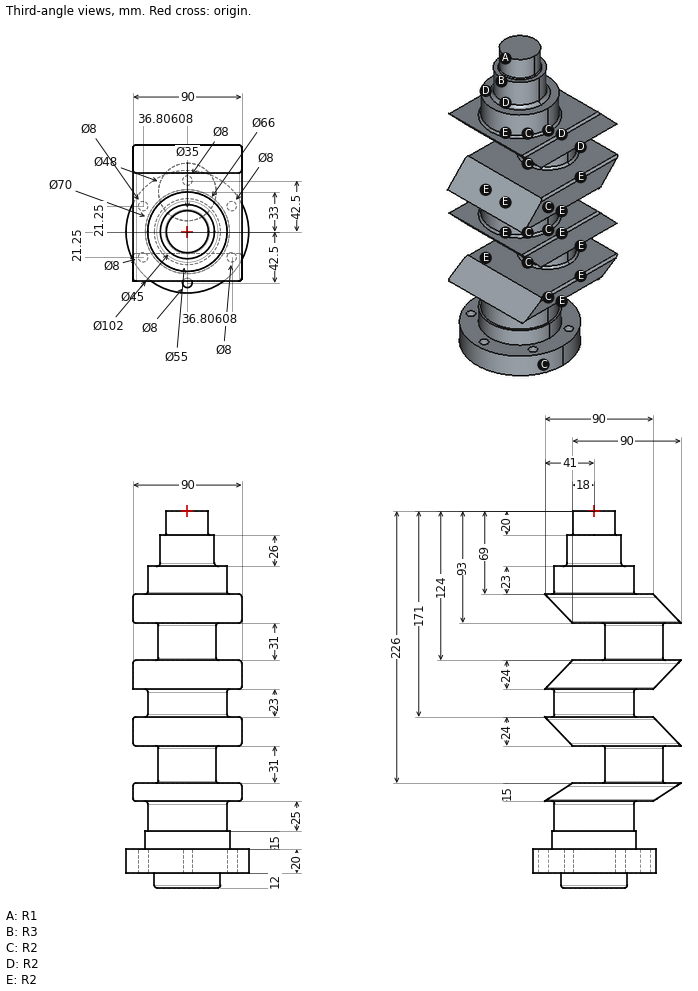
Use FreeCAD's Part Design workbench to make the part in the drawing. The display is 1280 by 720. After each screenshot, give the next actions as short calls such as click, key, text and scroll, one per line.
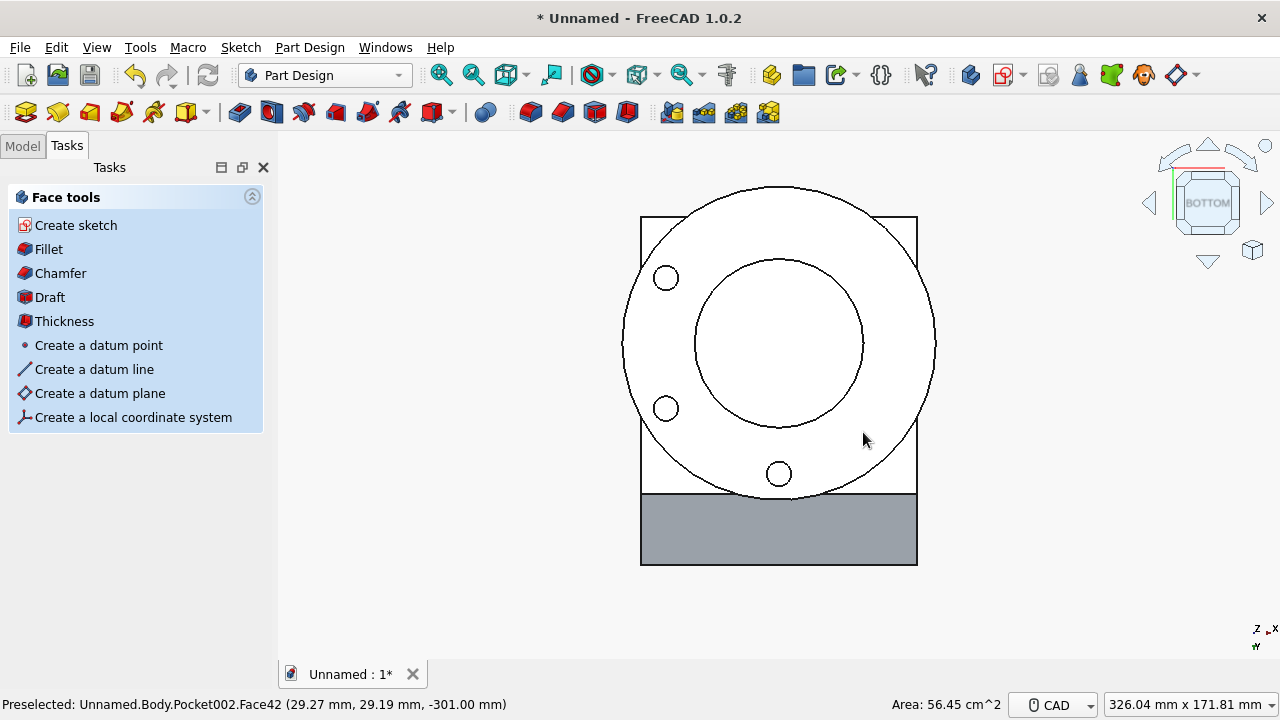
click(1004, 76)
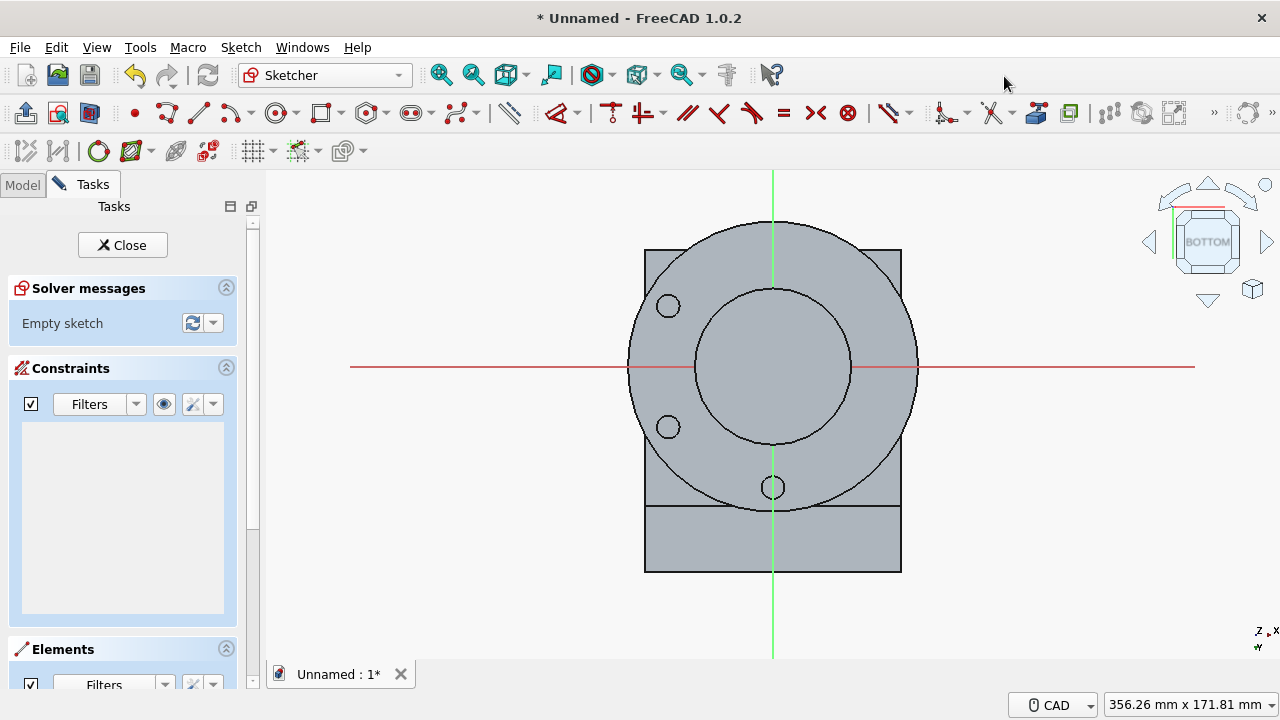
click(90, 114)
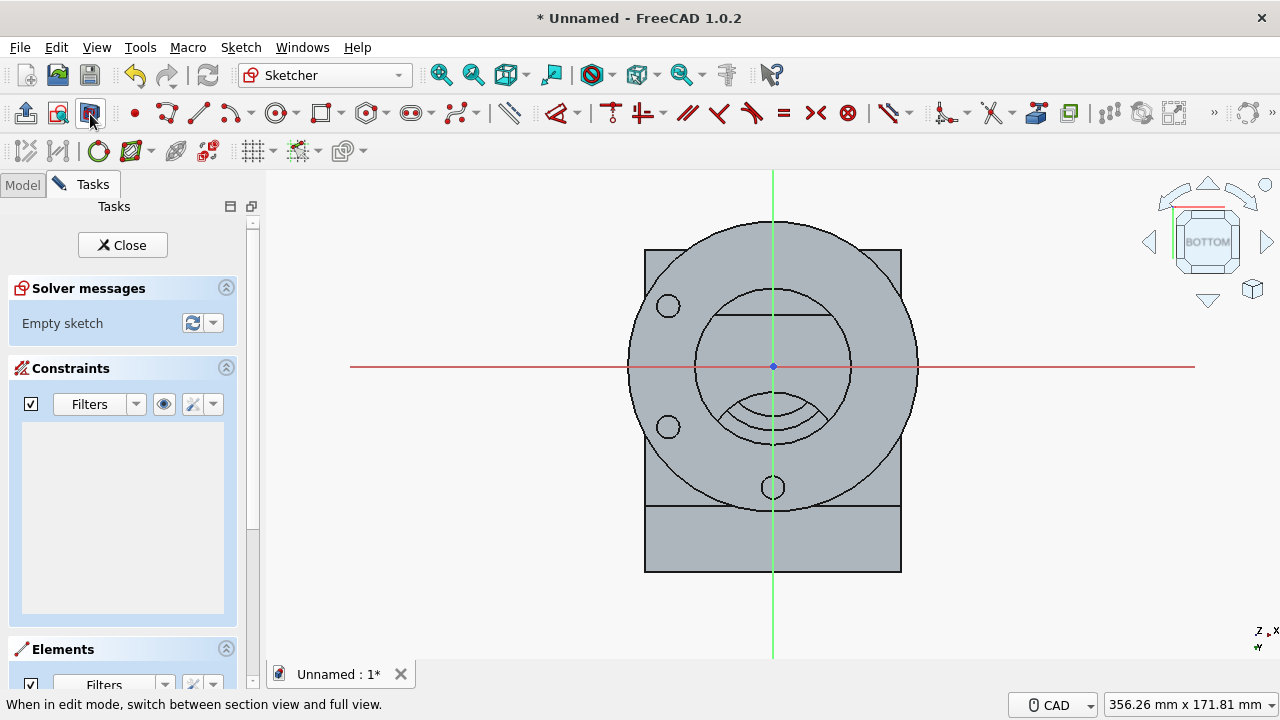
scroll(779, 232, up, 13)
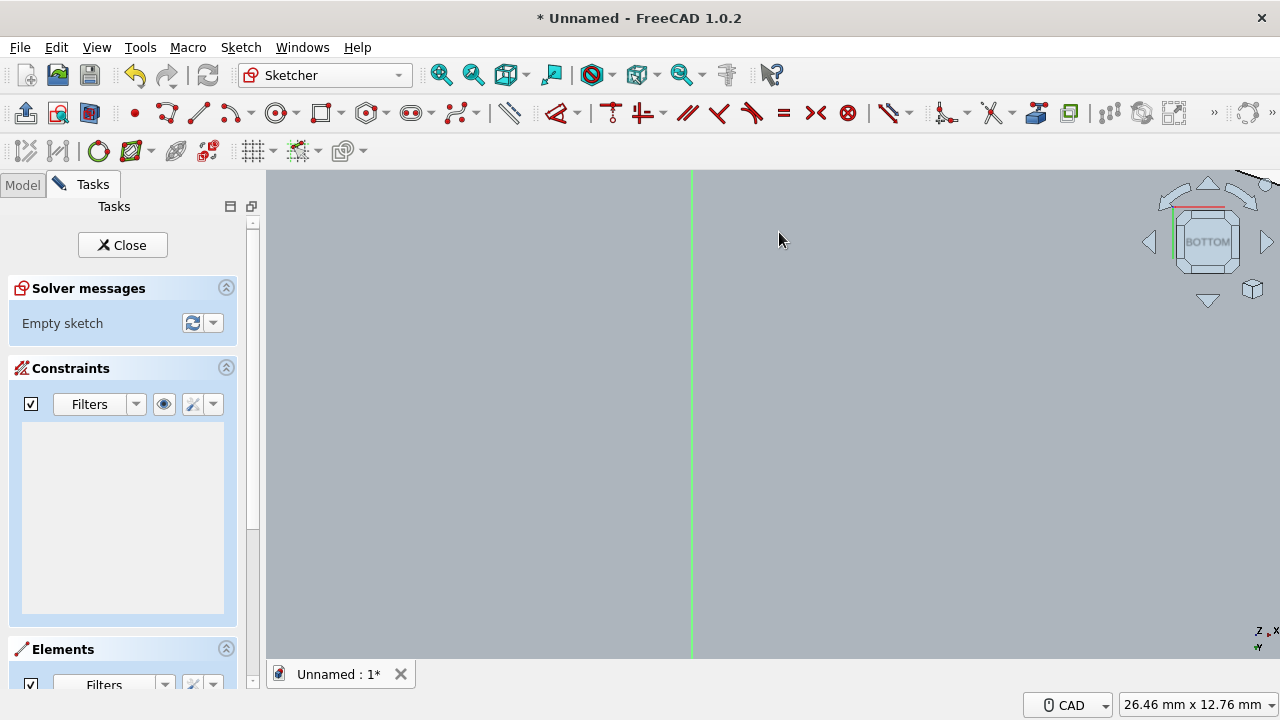
click(276, 114)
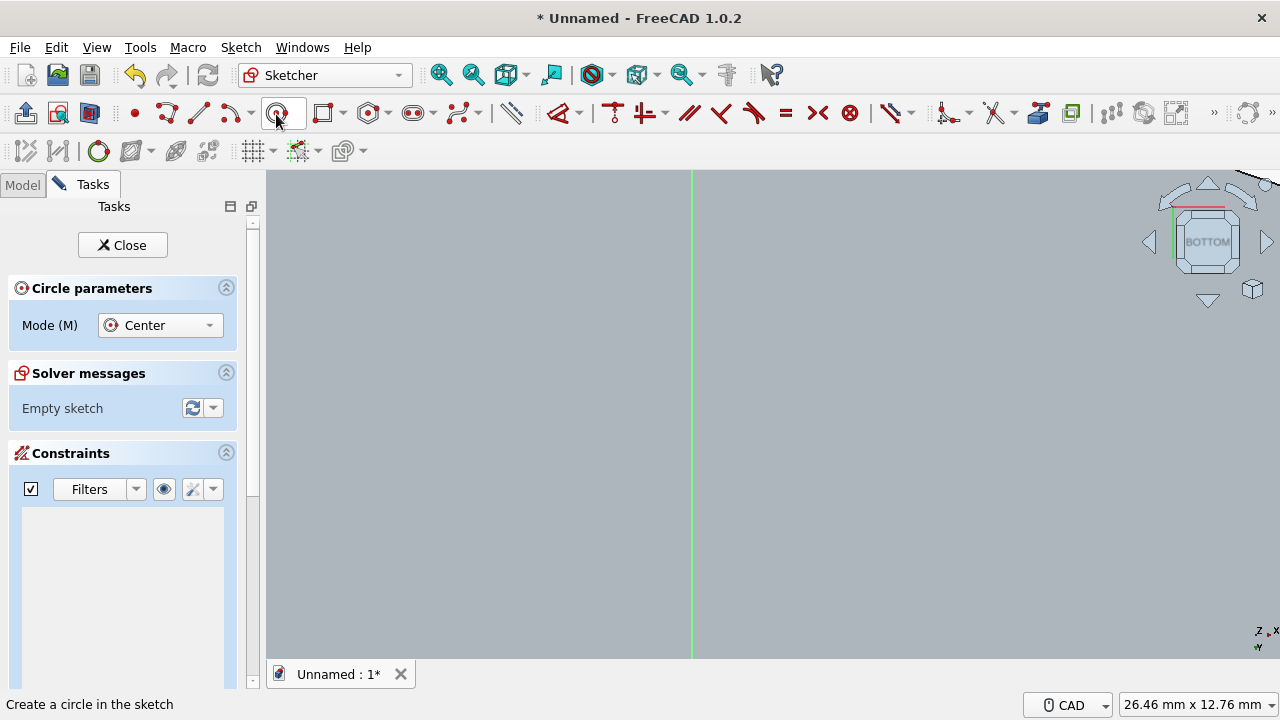
click(692, 414)
move(801, 306)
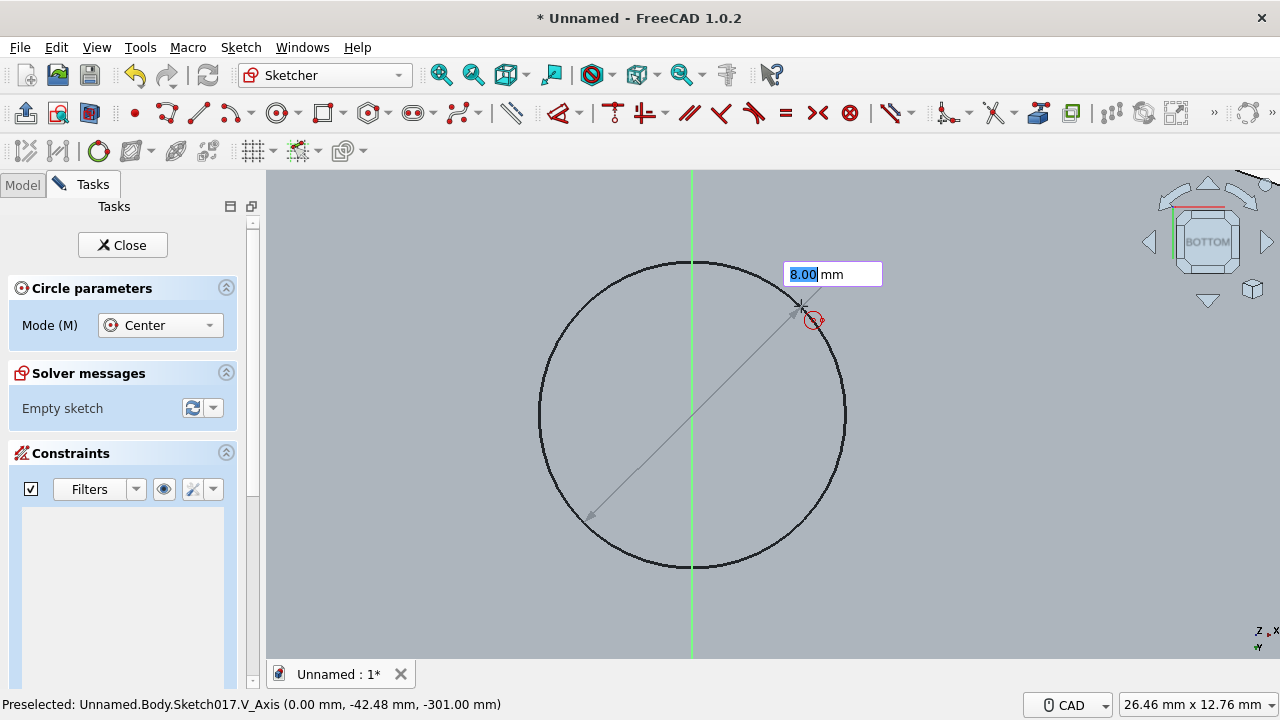
text(8)
key(Return)
key(Escape)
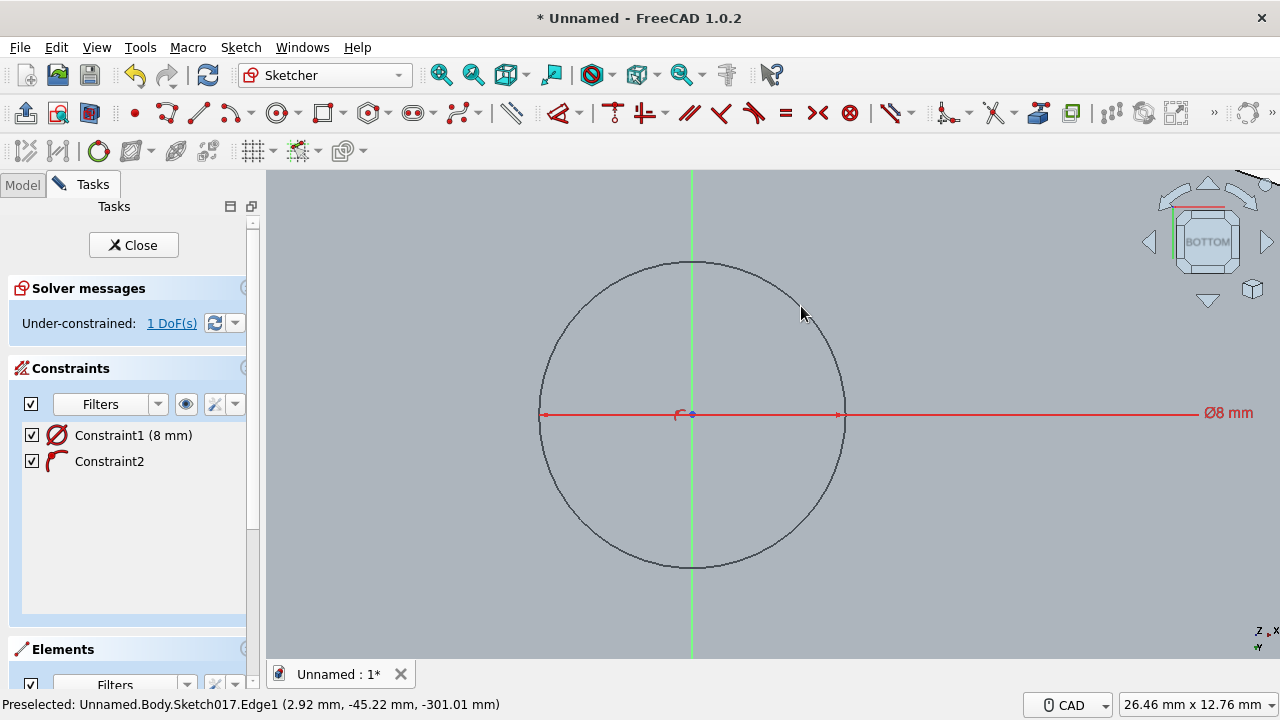
click(558, 114)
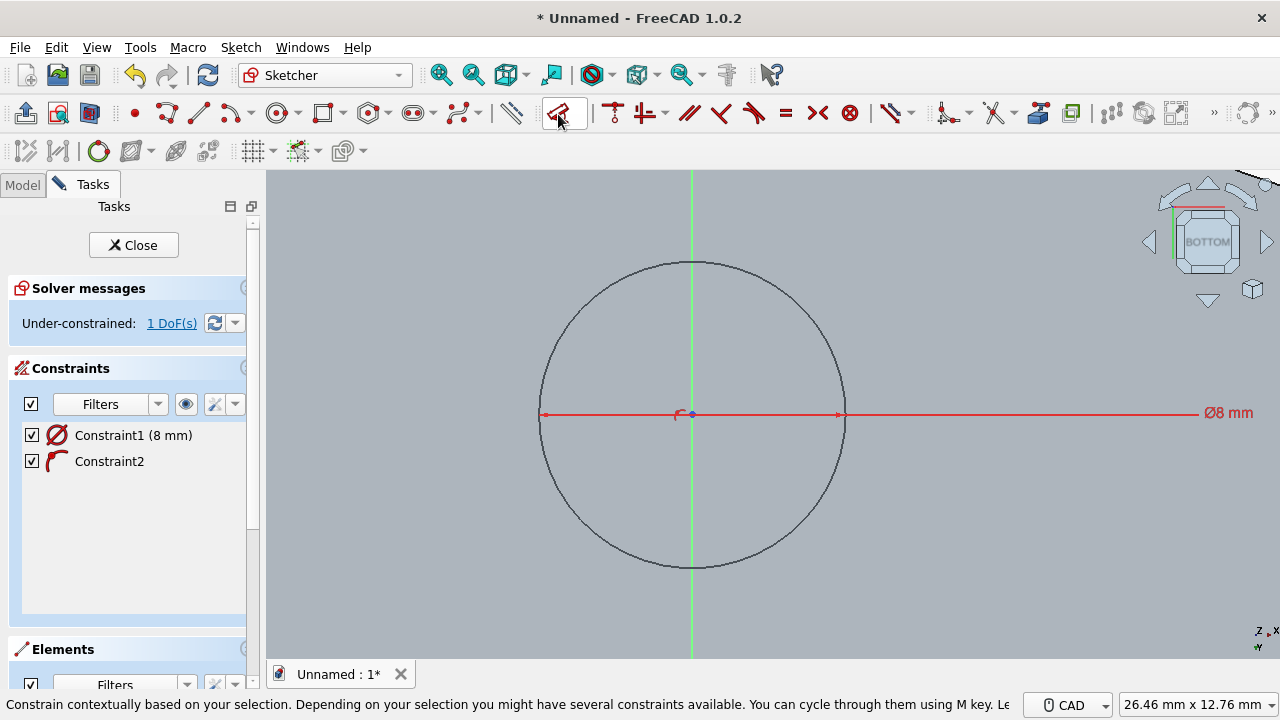
click(692, 415)
click(726, 523)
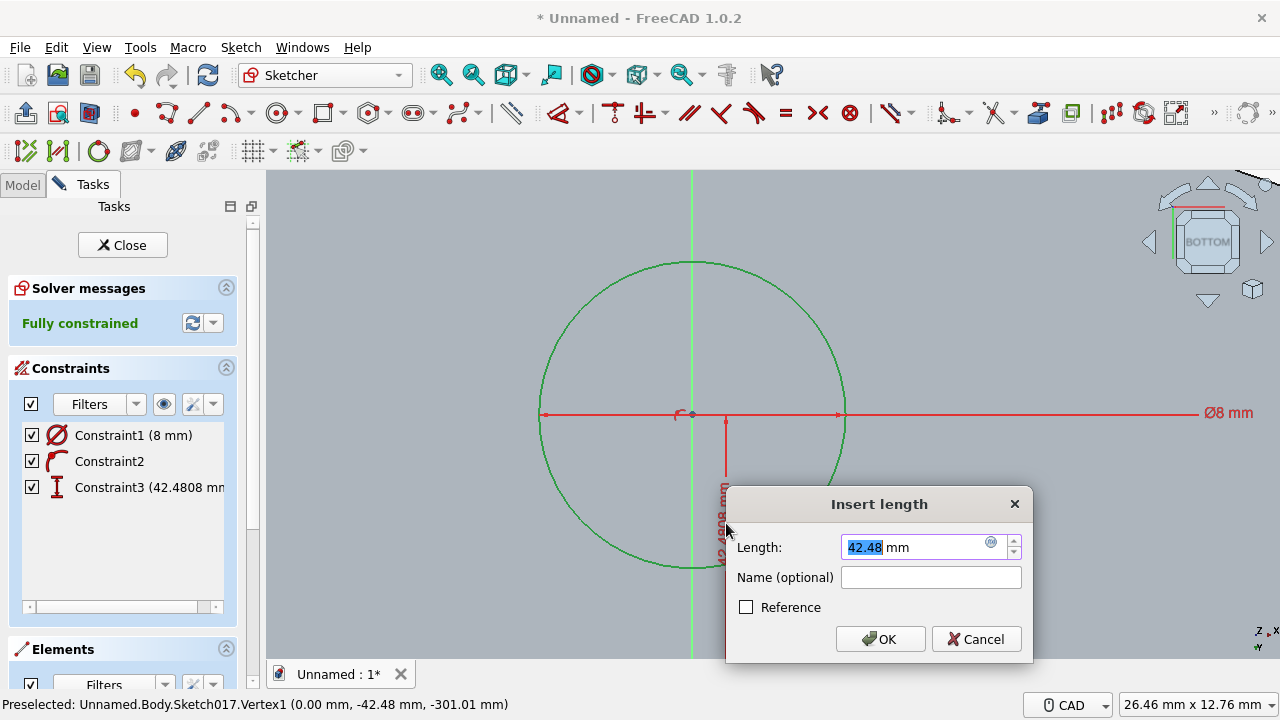
text(42.5)
key(Return)
key(Escape)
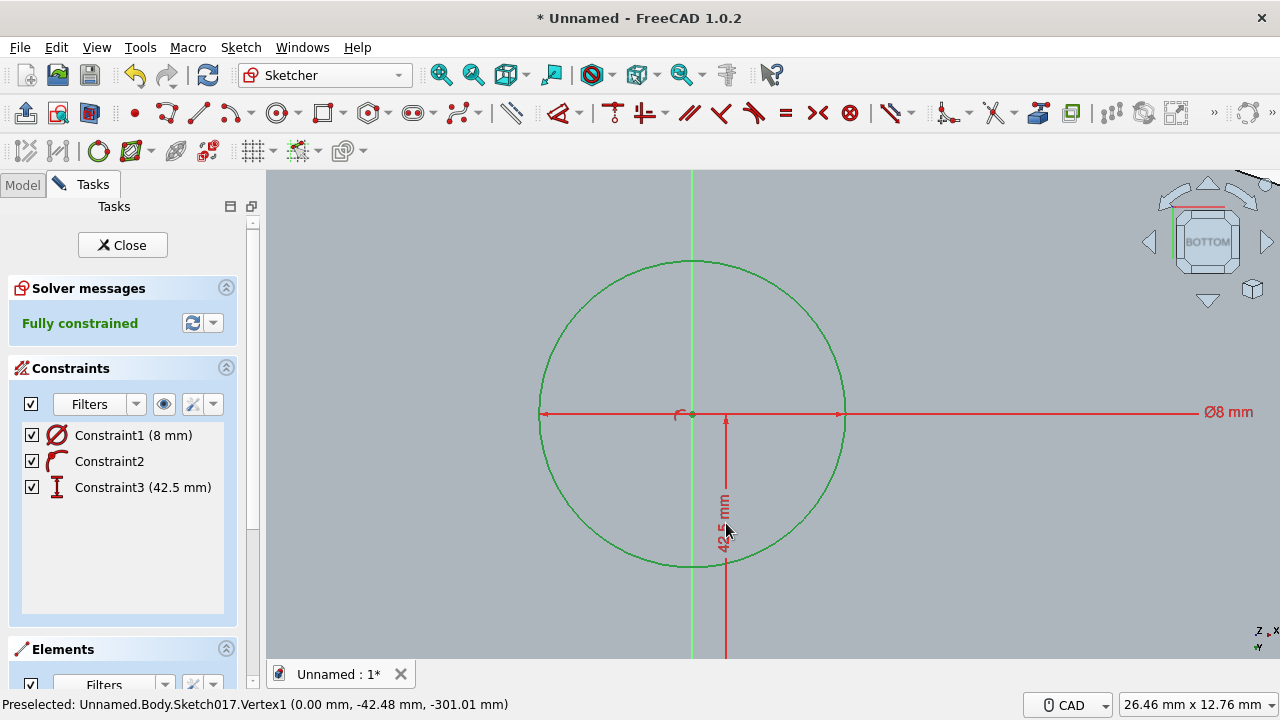
click(123, 245)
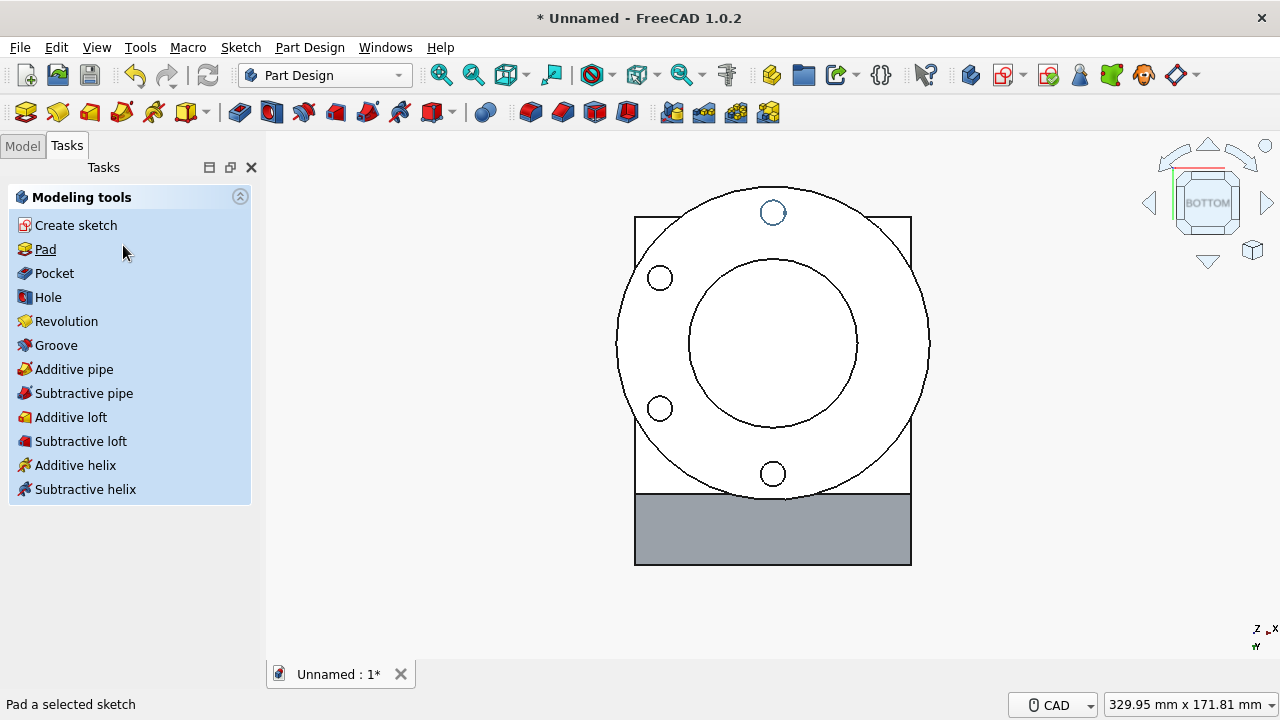
click(240, 112)